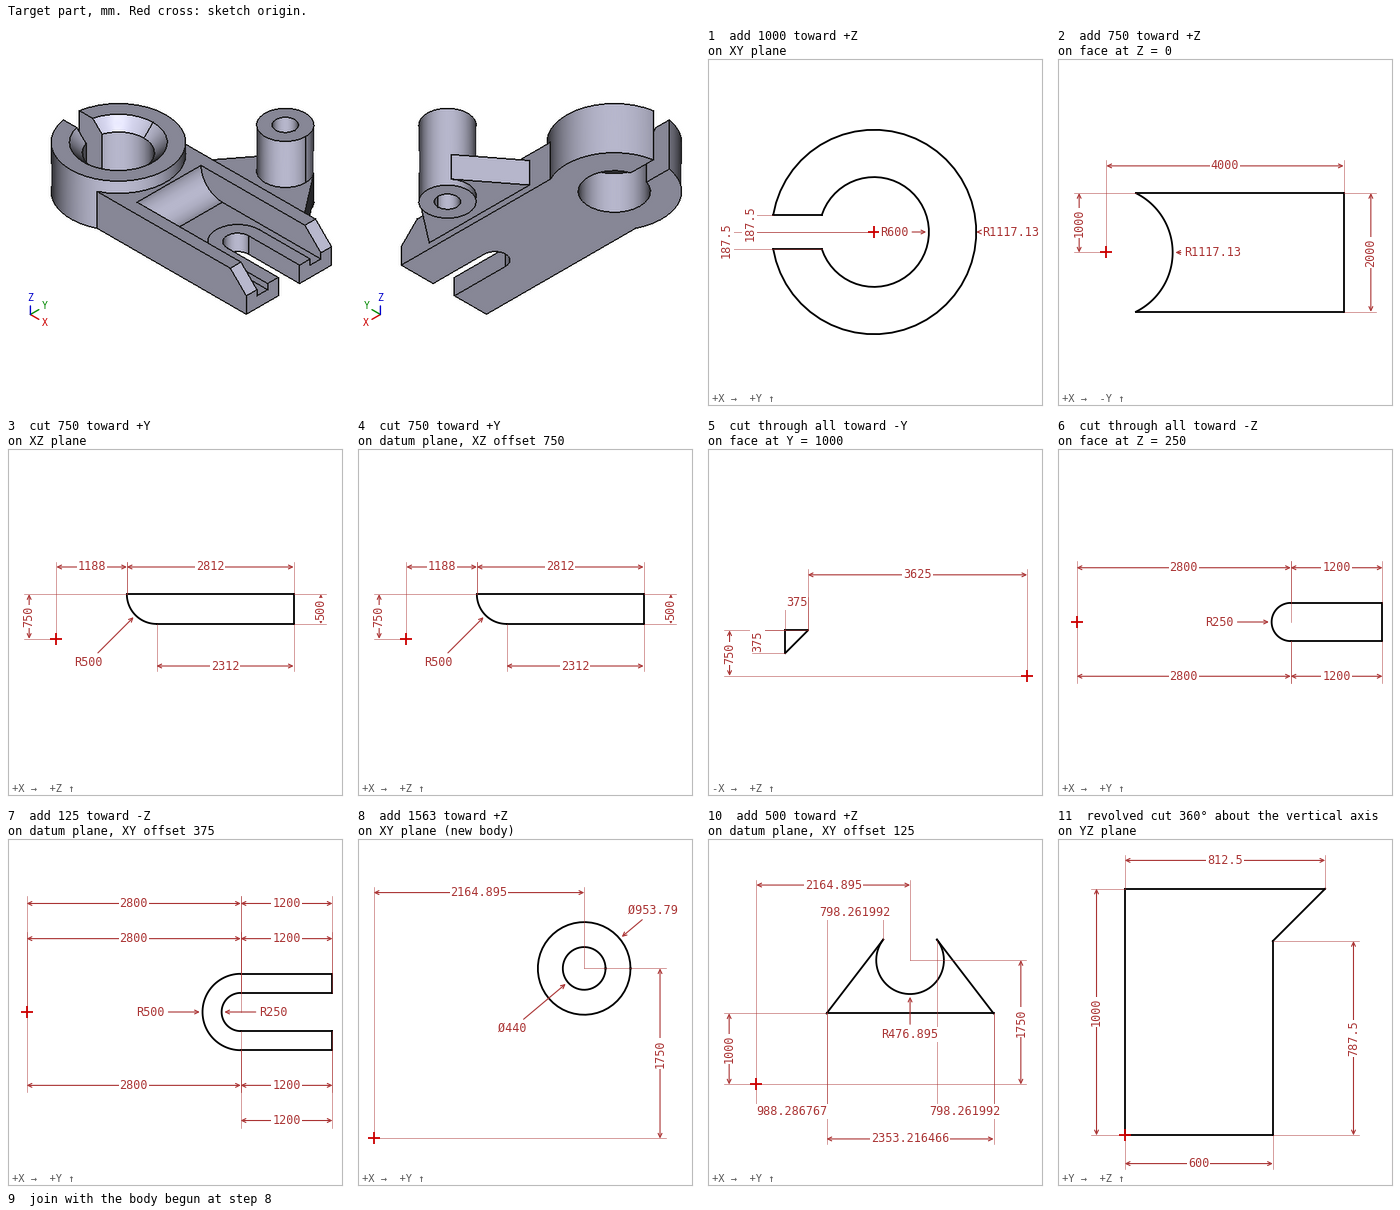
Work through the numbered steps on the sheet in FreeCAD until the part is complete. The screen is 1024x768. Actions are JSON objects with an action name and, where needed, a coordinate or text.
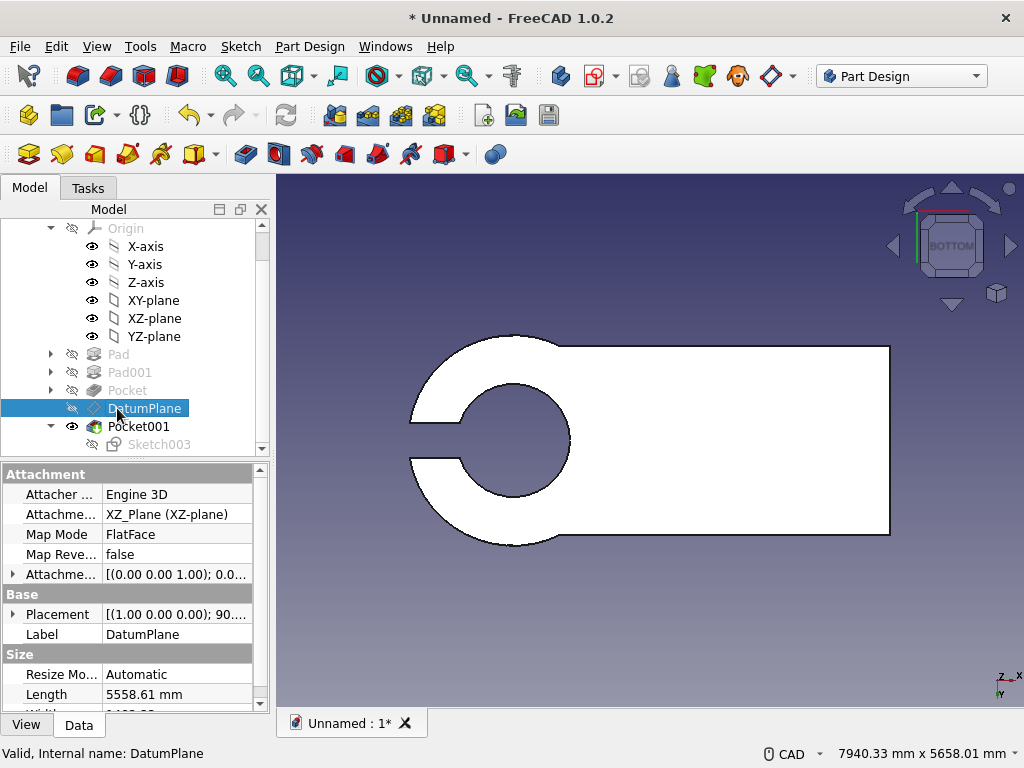
{"action": "key", "text": "4"}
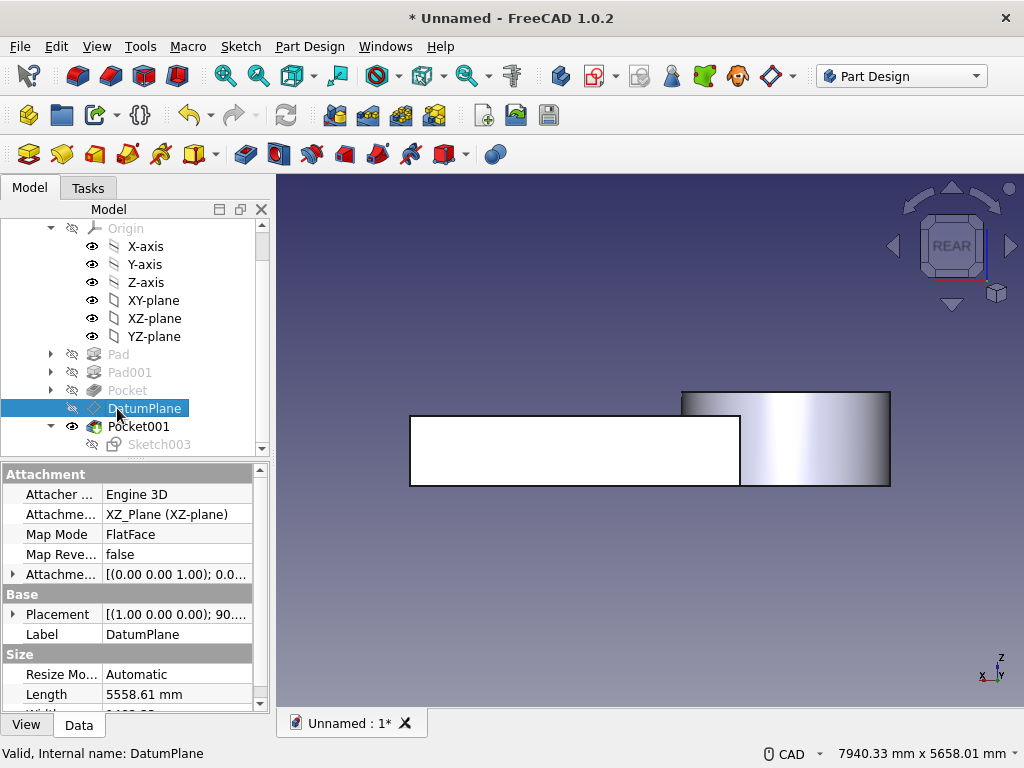
{"action": "left_click", "coordinate": [480, 450]}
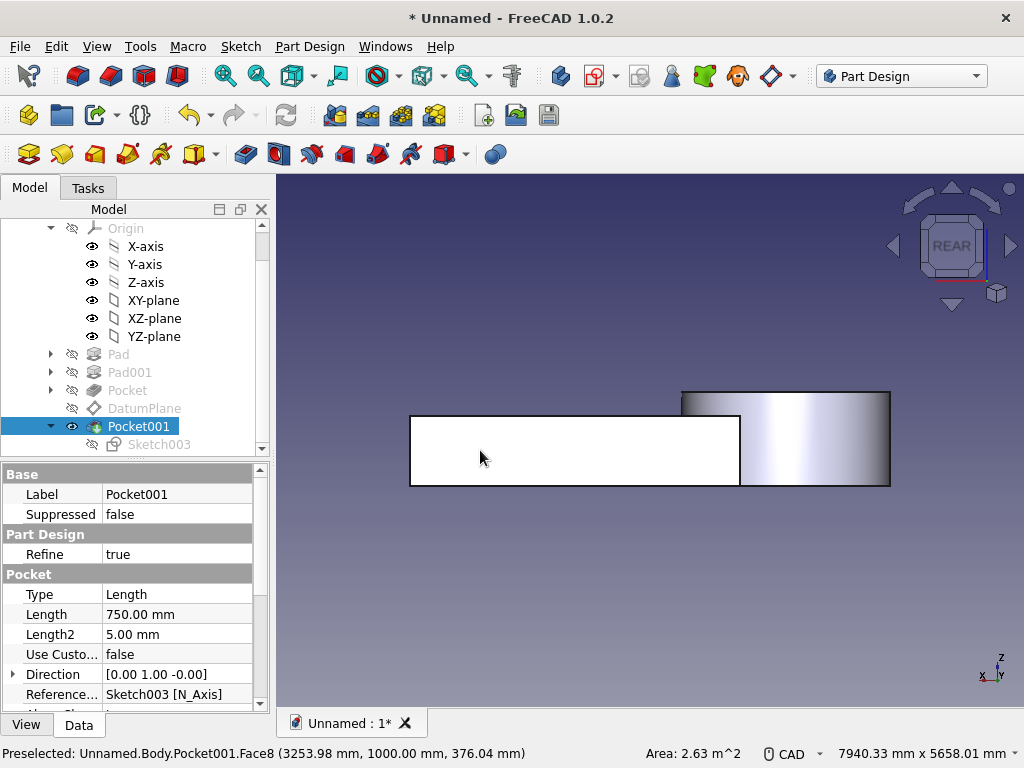
{"action": "left_click", "coordinate": [594, 76]}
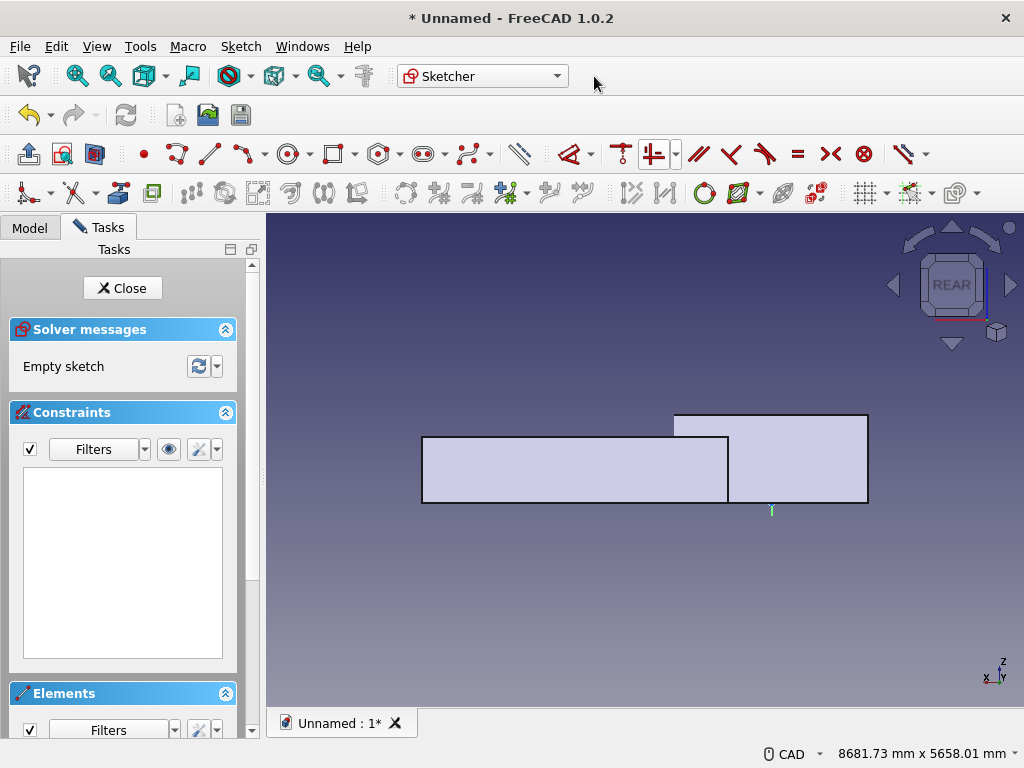
{"action": "scroll", "coordinate": [422, 453], "scroll_direction": "up", "scroll_amount": 11}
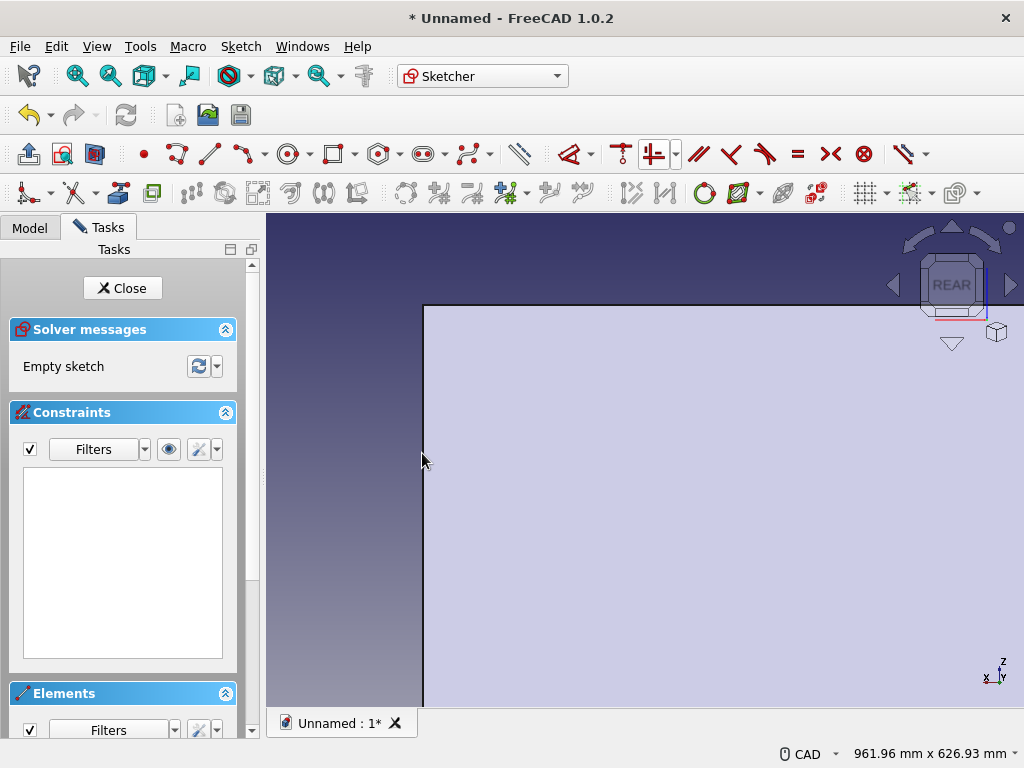
{"action": "key", "text": "g m"}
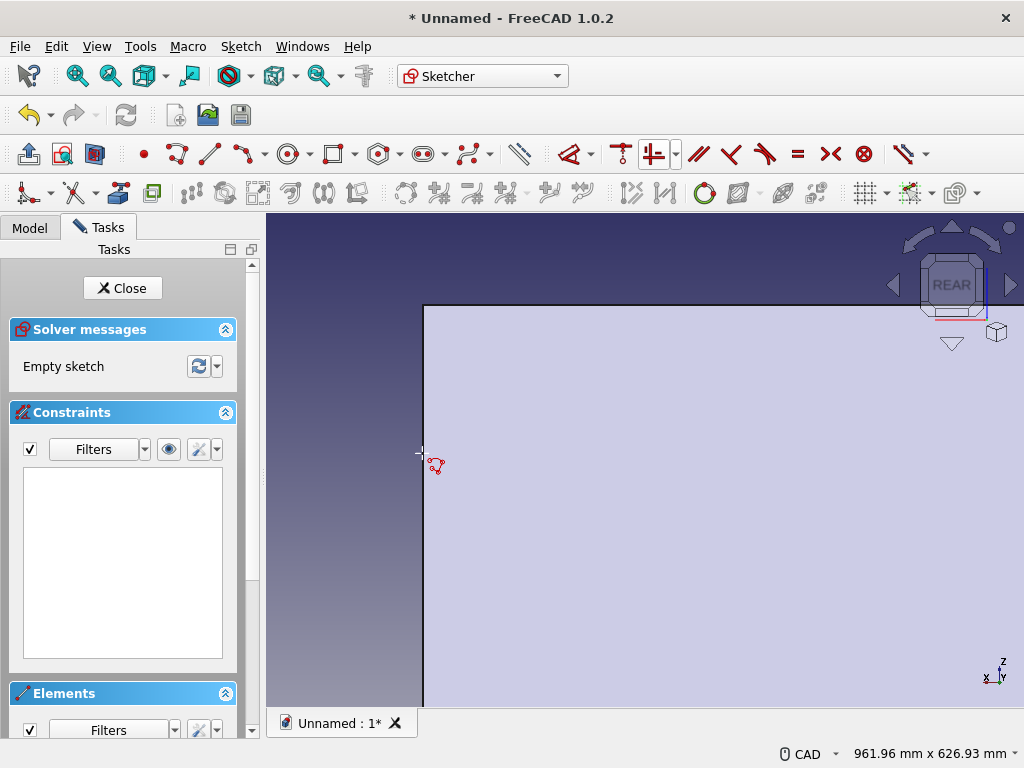
{"action": "left_click", "coordinate": [719, 305]}
{"action": "left_click", "coordinate": [423, 305]}
{"action": "left_click", "coordinate": [423, 601]}
{"action": "left_click", "coordinate": [719, 306]}
{"action": "key", "text": "Escape"}
{"action": "key", "text": "Escape"}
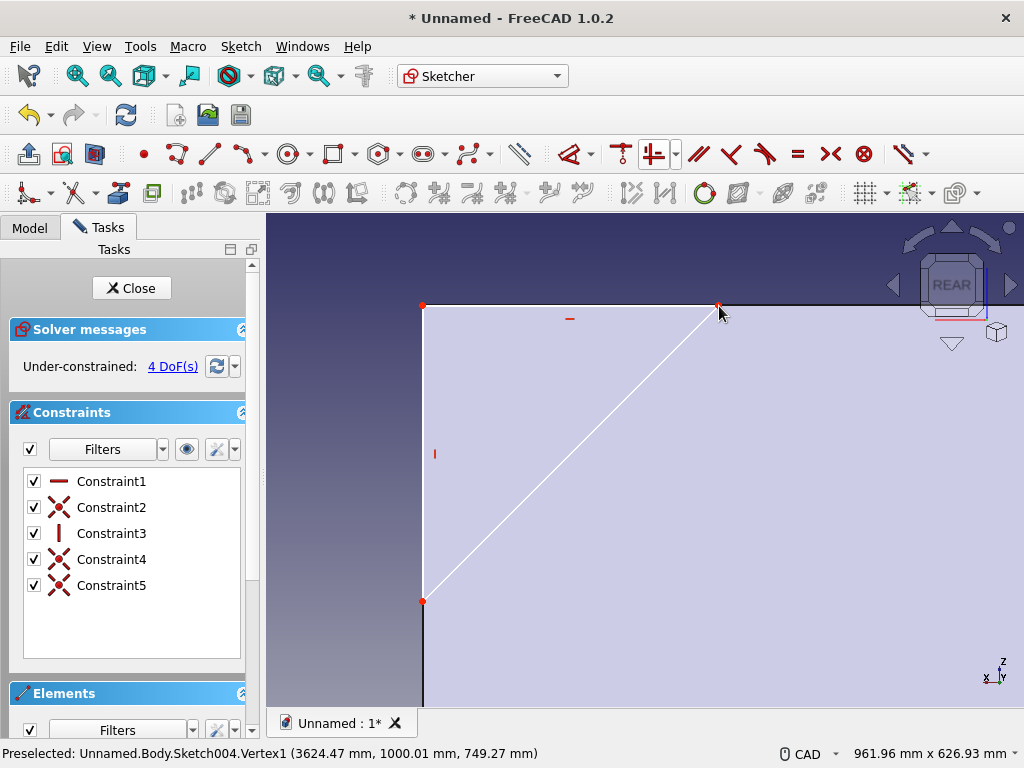
{"action": "key", "text": "d"}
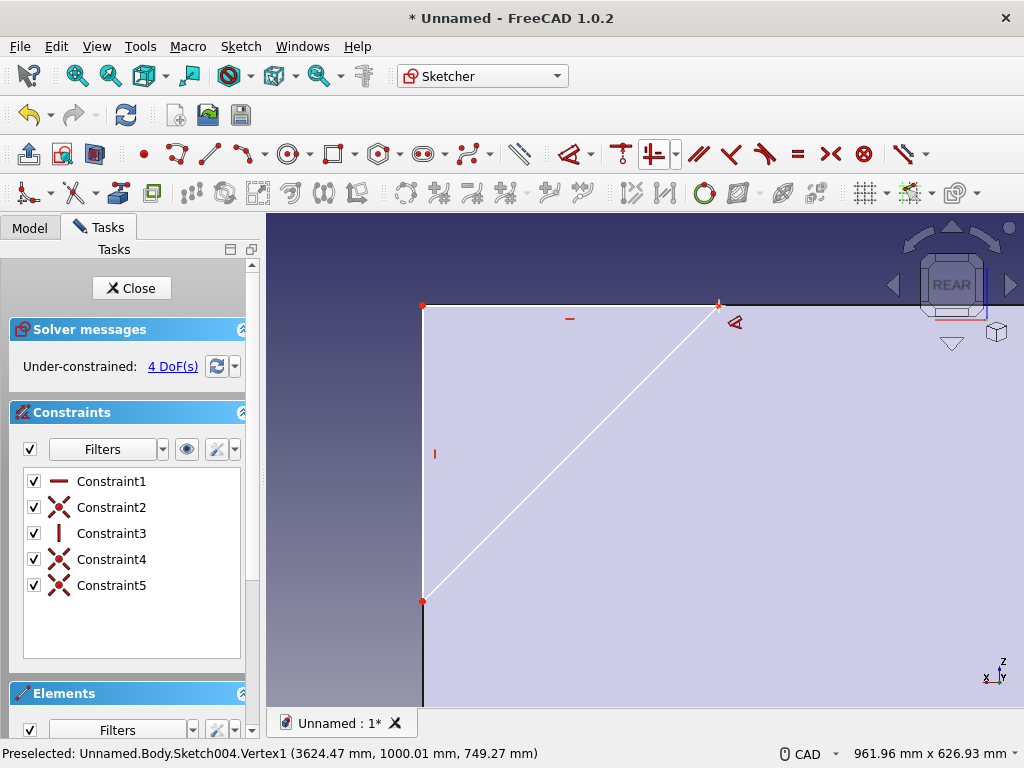
{"action": "left_click", "coordinate": [630, 306]}
{"action": "left_click", "coordinate": [571, 272]}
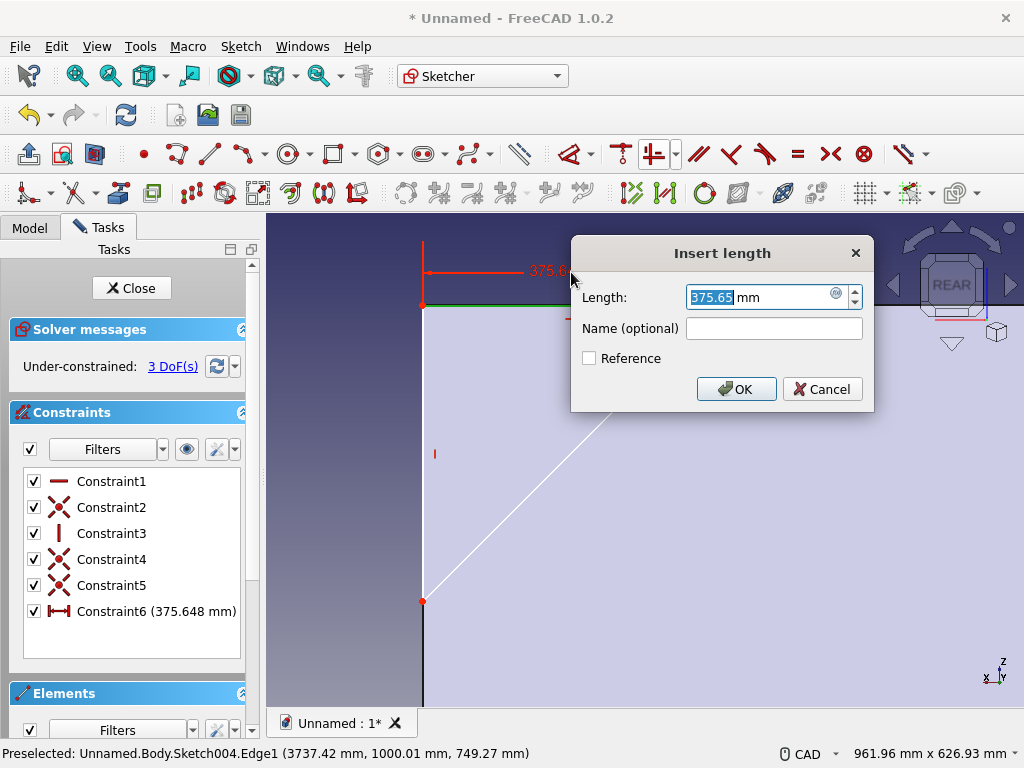
{"action": "type", "text": "375"}
{"action": "key", "text": "Return"}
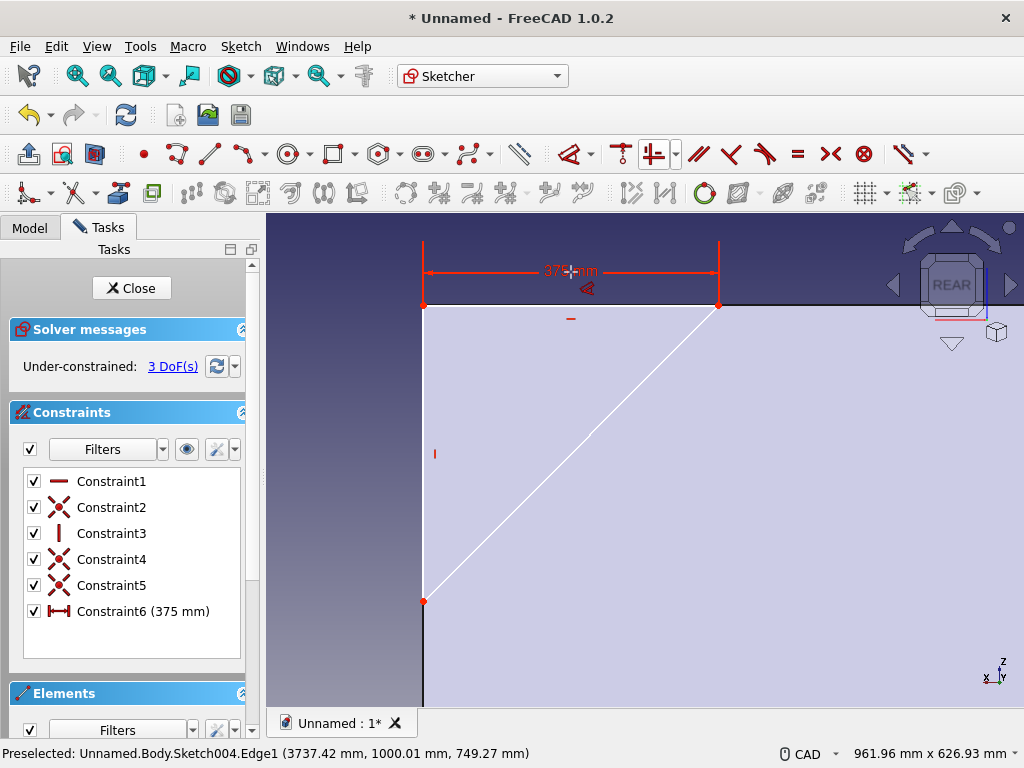
{"action": "left_click", "coordinate": [423, 395]}
{"action": "left_click", "coordinate": [389, 454]}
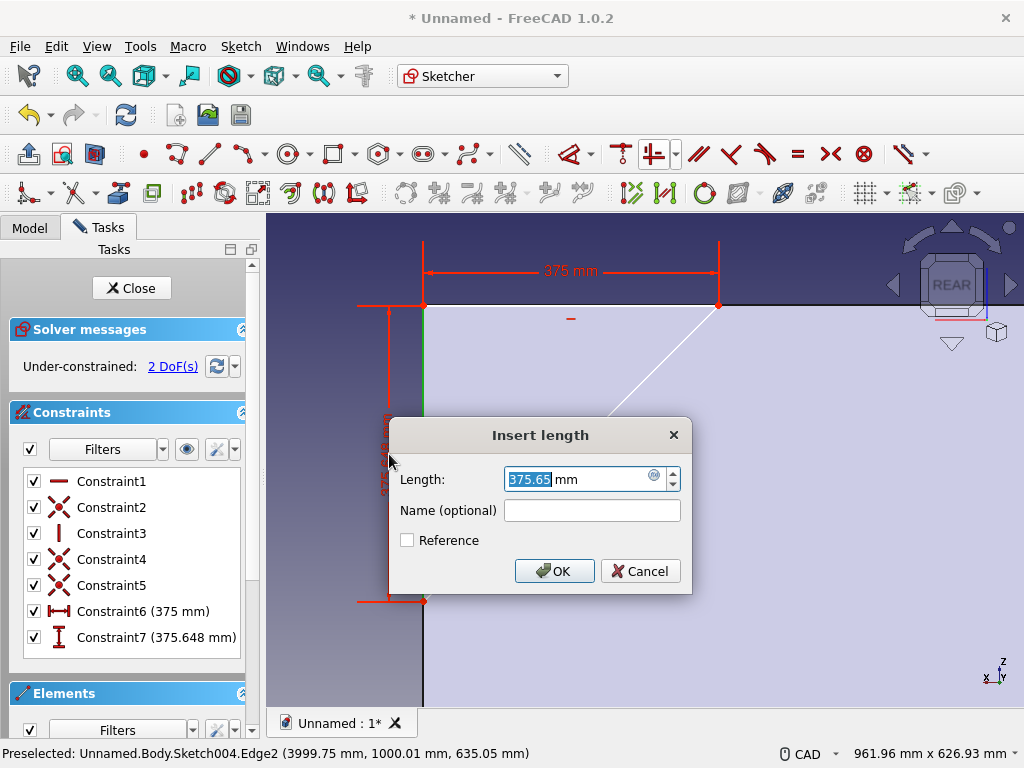
{"action": "type", "text": "375"}
{"action": "key", "text": "Return"}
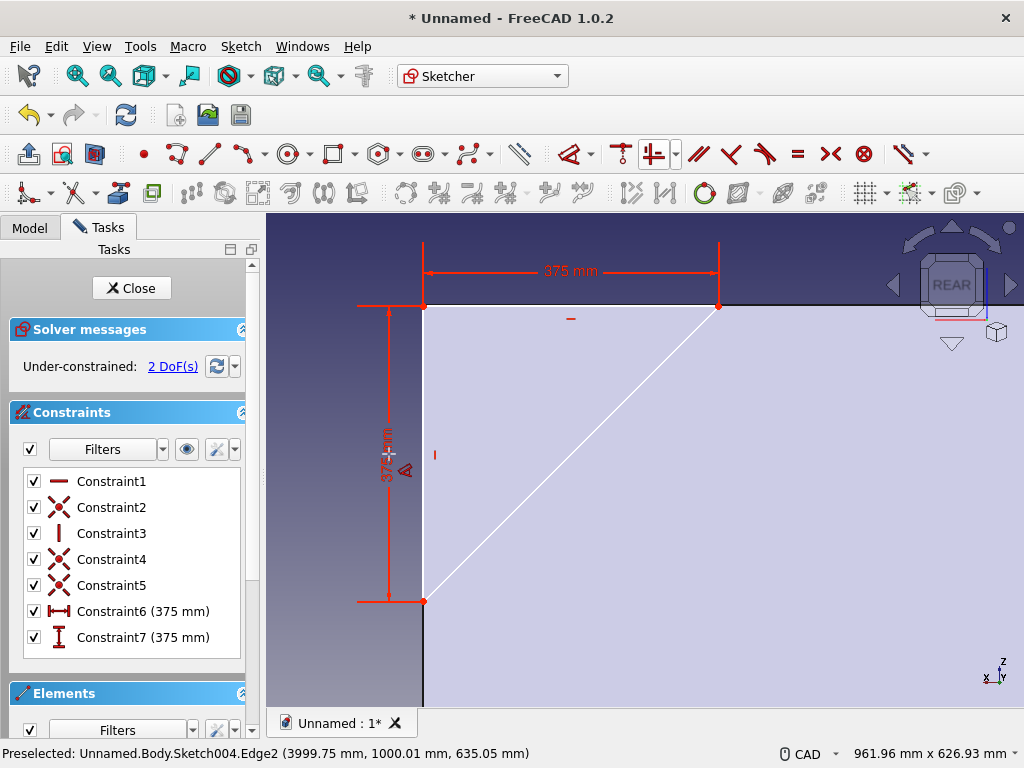
{"action": "left_click", "coordinate": [719, 306]}
{"action": "left_click", "coordinate": [685, 493]}